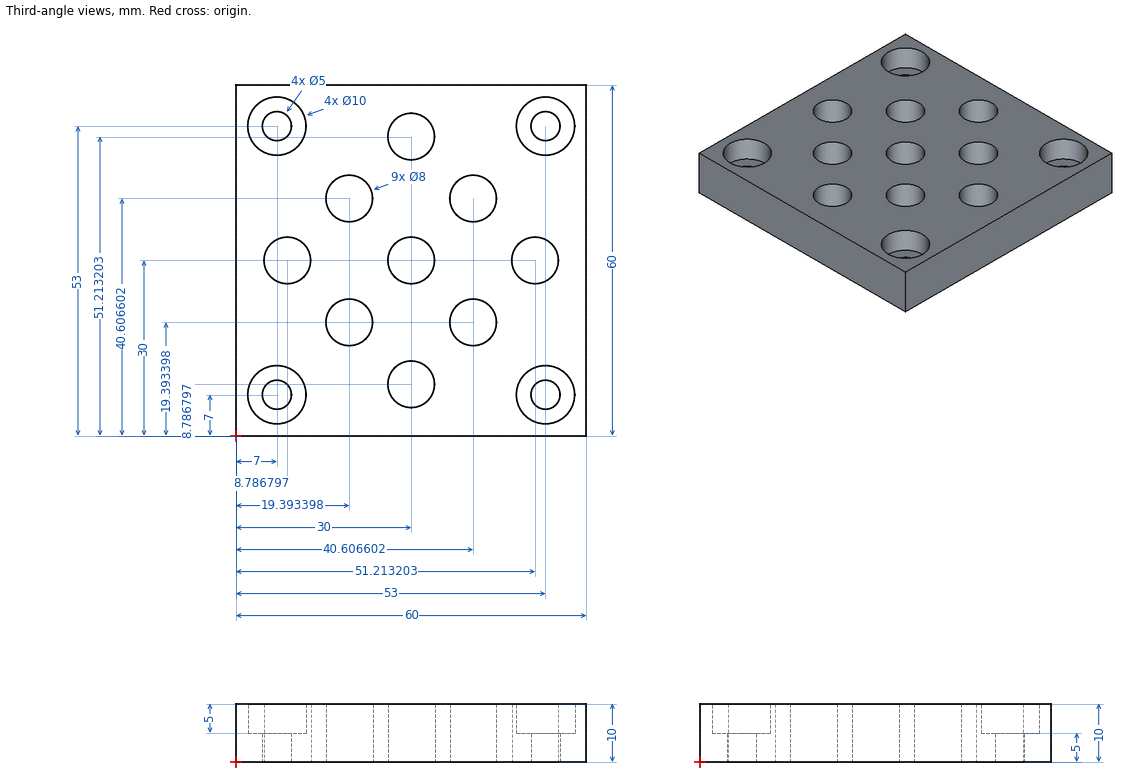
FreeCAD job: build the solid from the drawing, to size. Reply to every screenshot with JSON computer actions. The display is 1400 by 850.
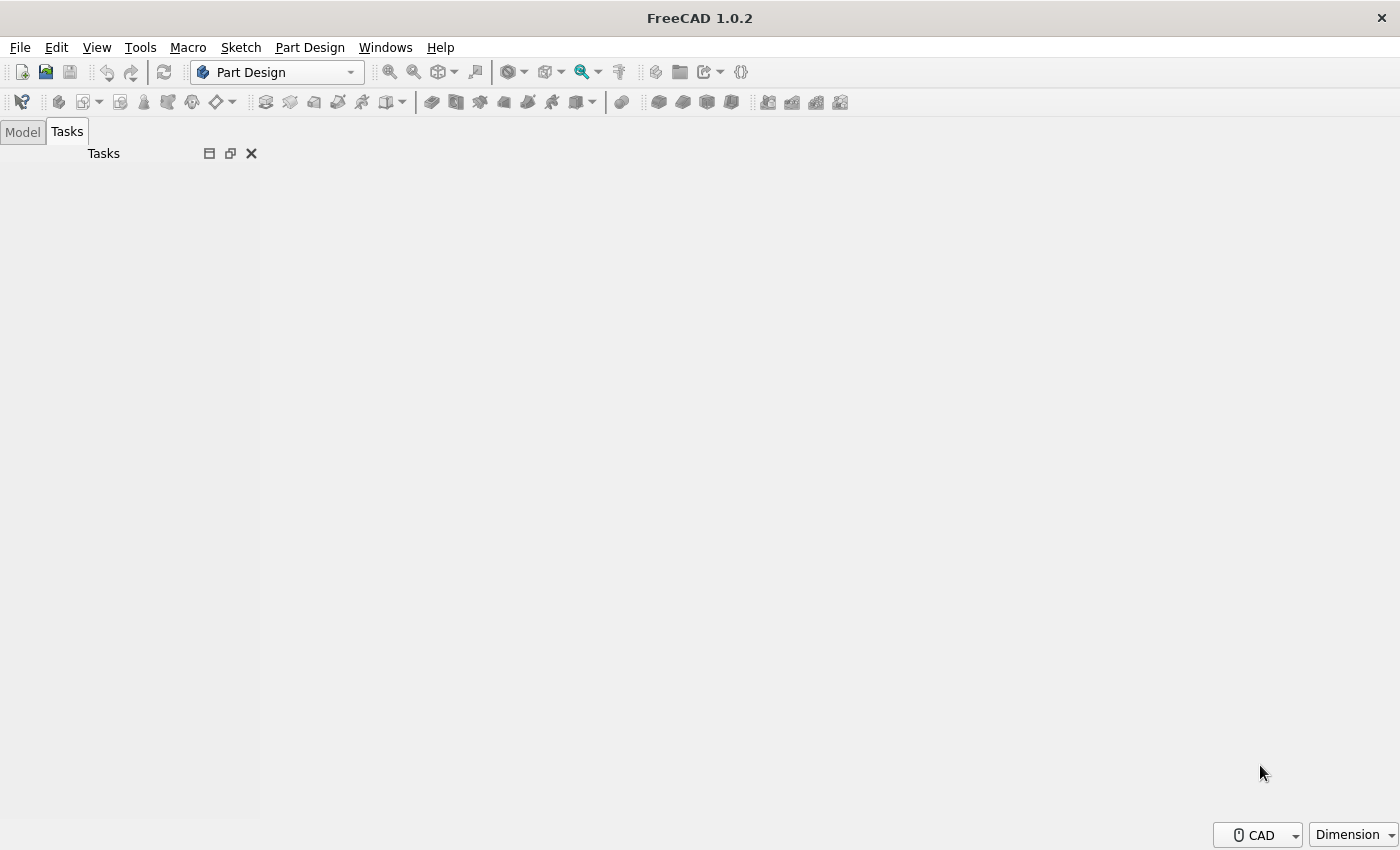
{"action": "left_click", "coordinate": [22, 72]}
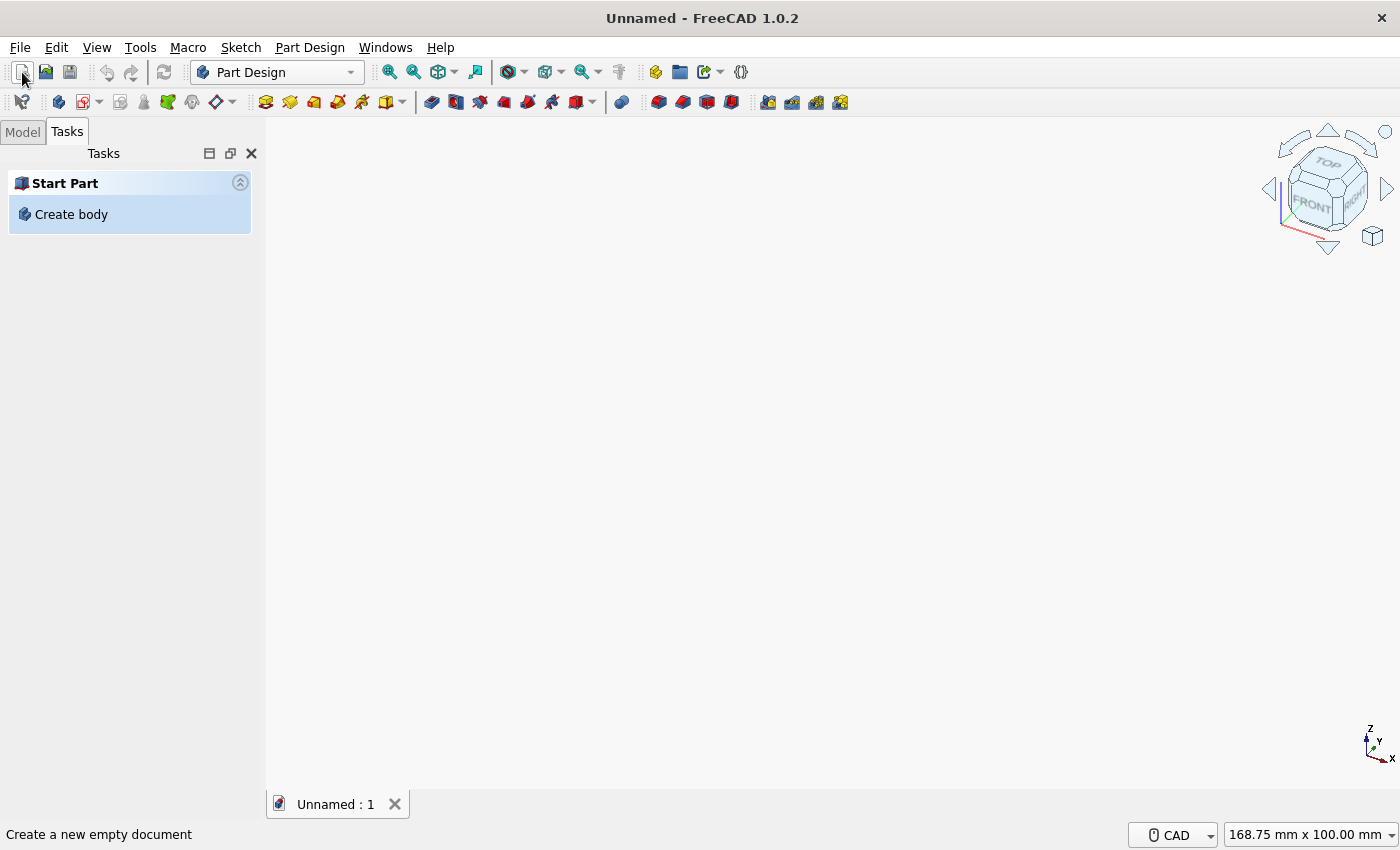
{"action": "left_click", "coordinate": [84, 102]}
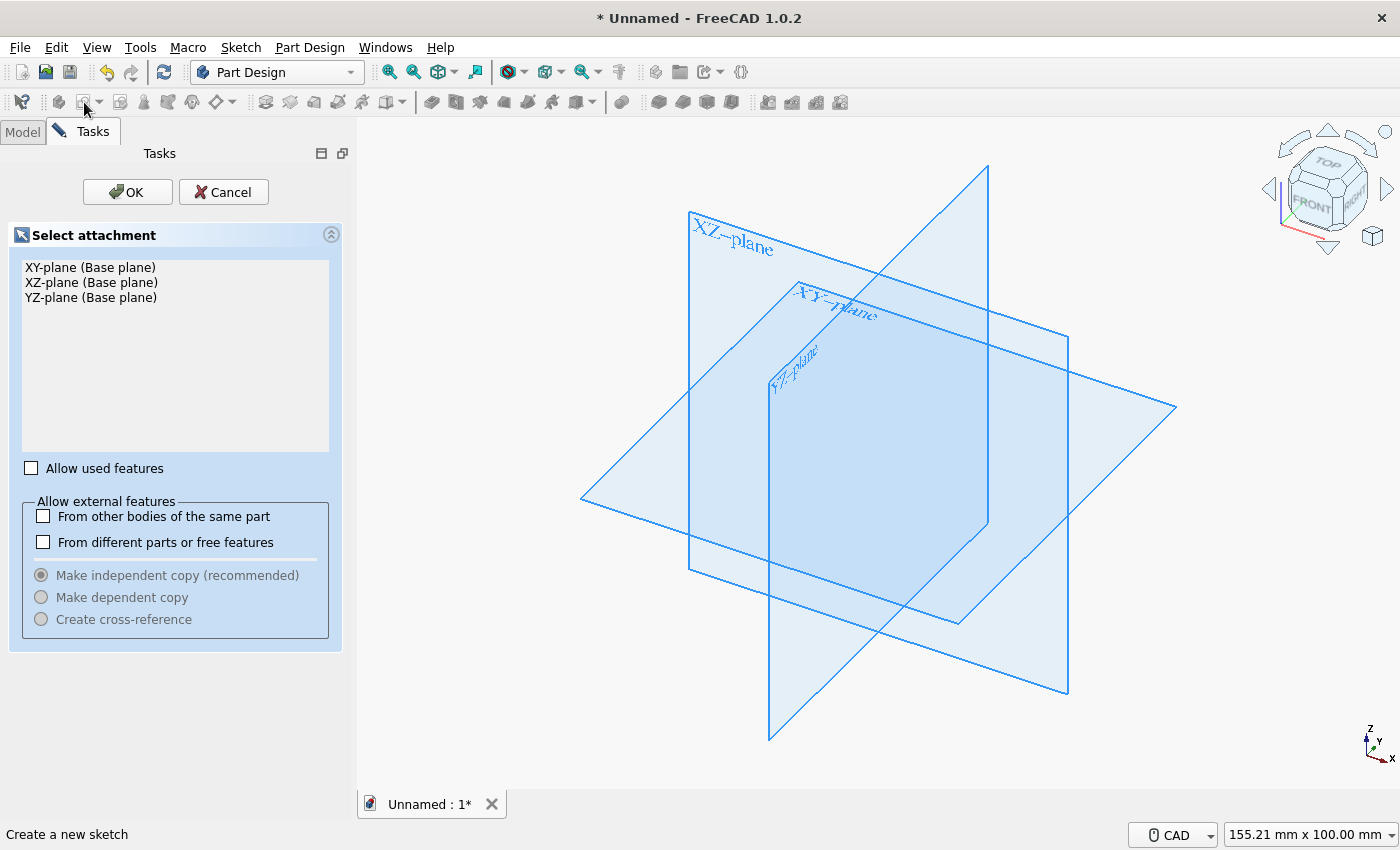
{"action": "left_click", "coordinate": [82, 268]}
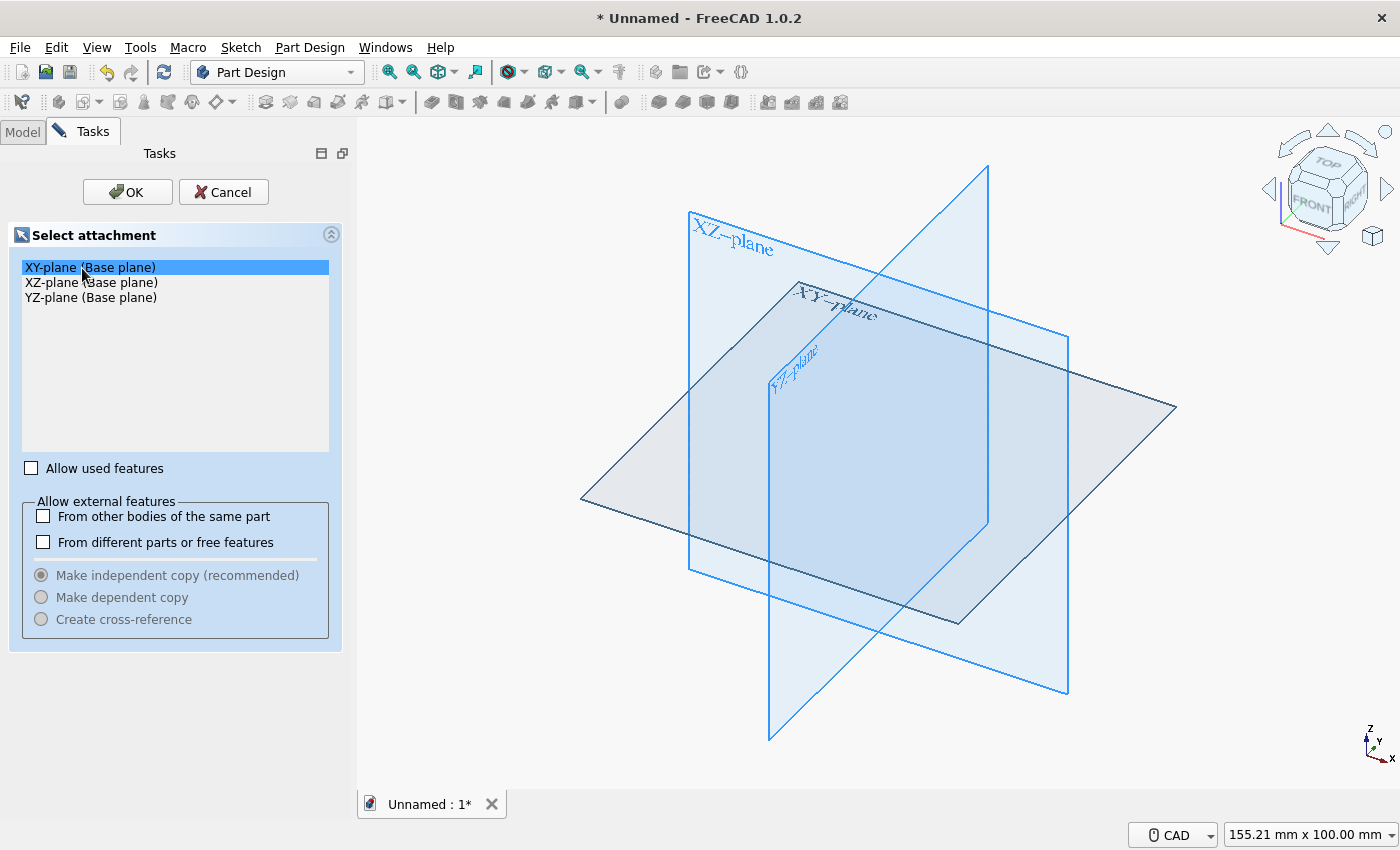
{"action": "left_click", "coordinate": [128, 192]}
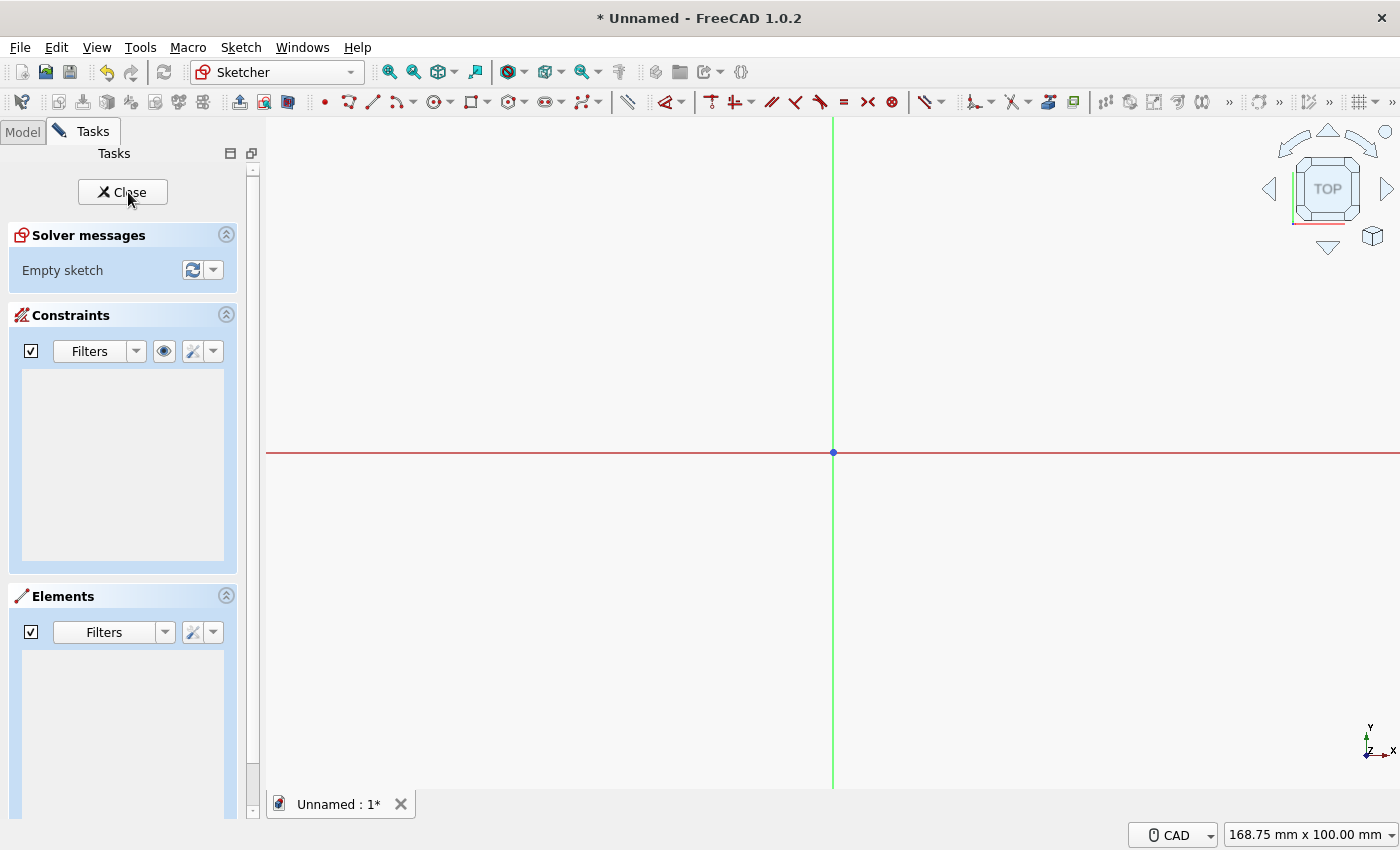
{"action": "scroll", "coordinate": [294, 761], "scroll_direction": "down", "scroll_amount": 1}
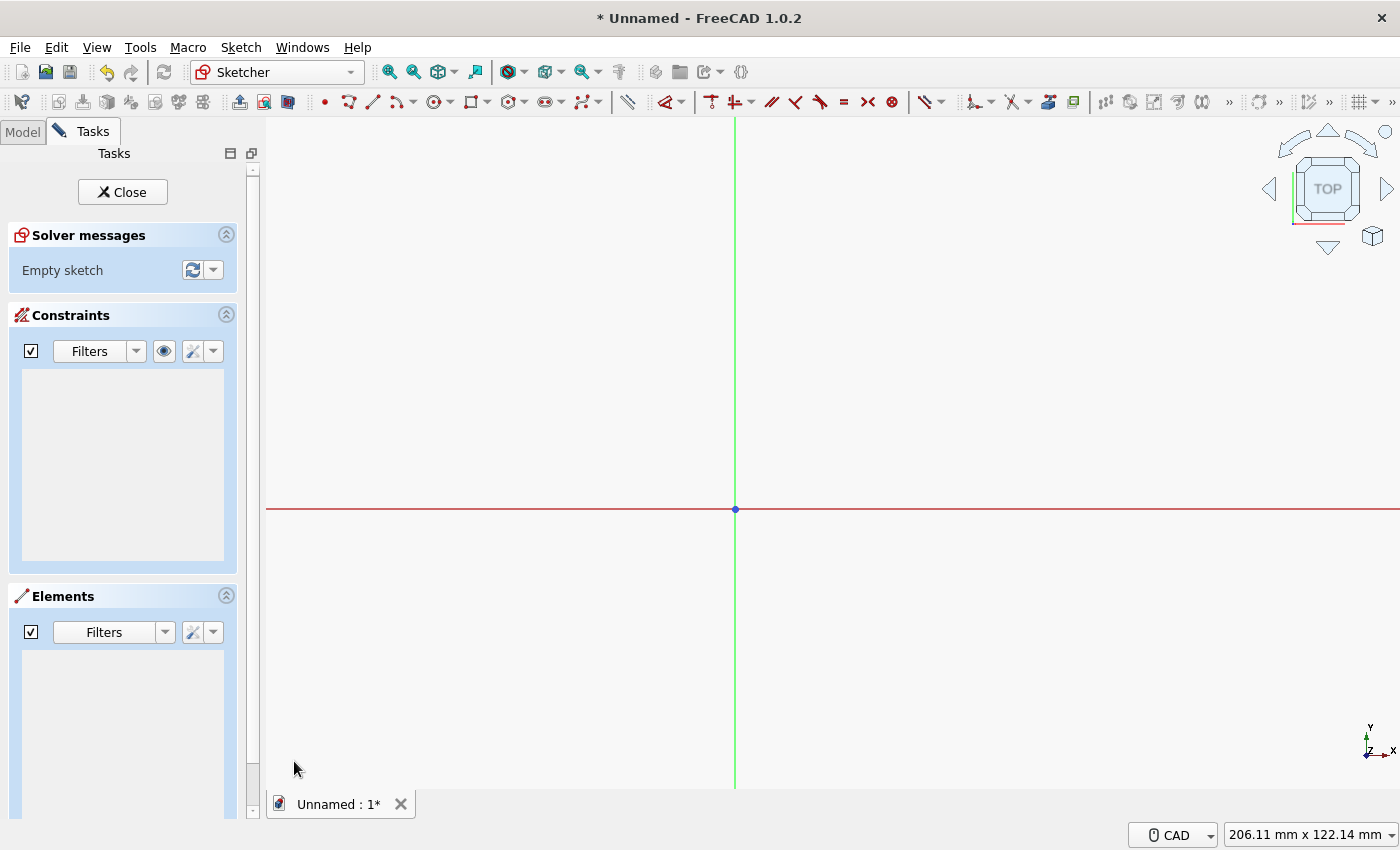
{"action": "left_click", "coordinate": [472, 102]}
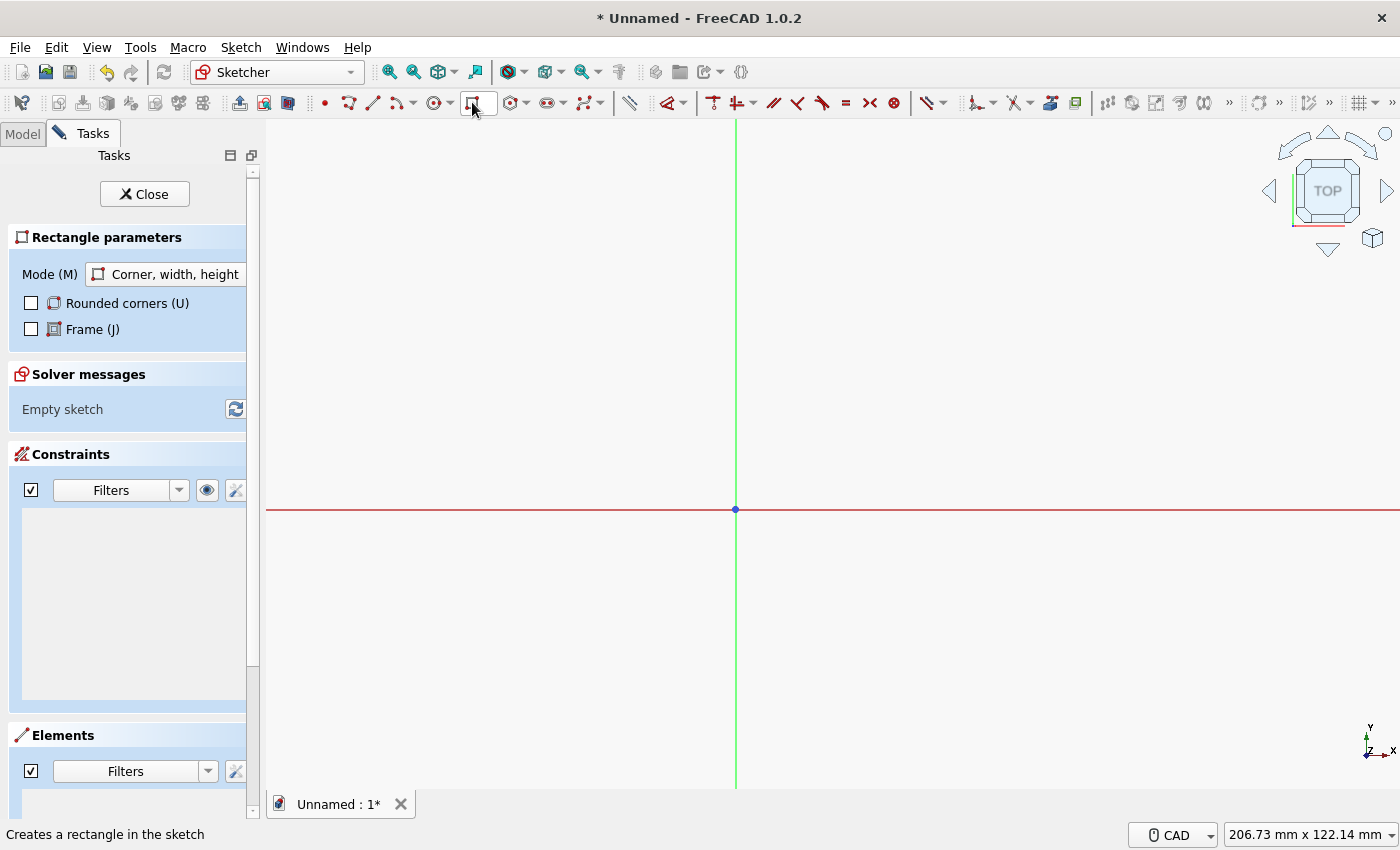
{"action": "left_click", "coordinate": [736, 510]}
{"action": "left_click", "coordinate": [1065, 181]}
{"action": "key", "text": "Escape"}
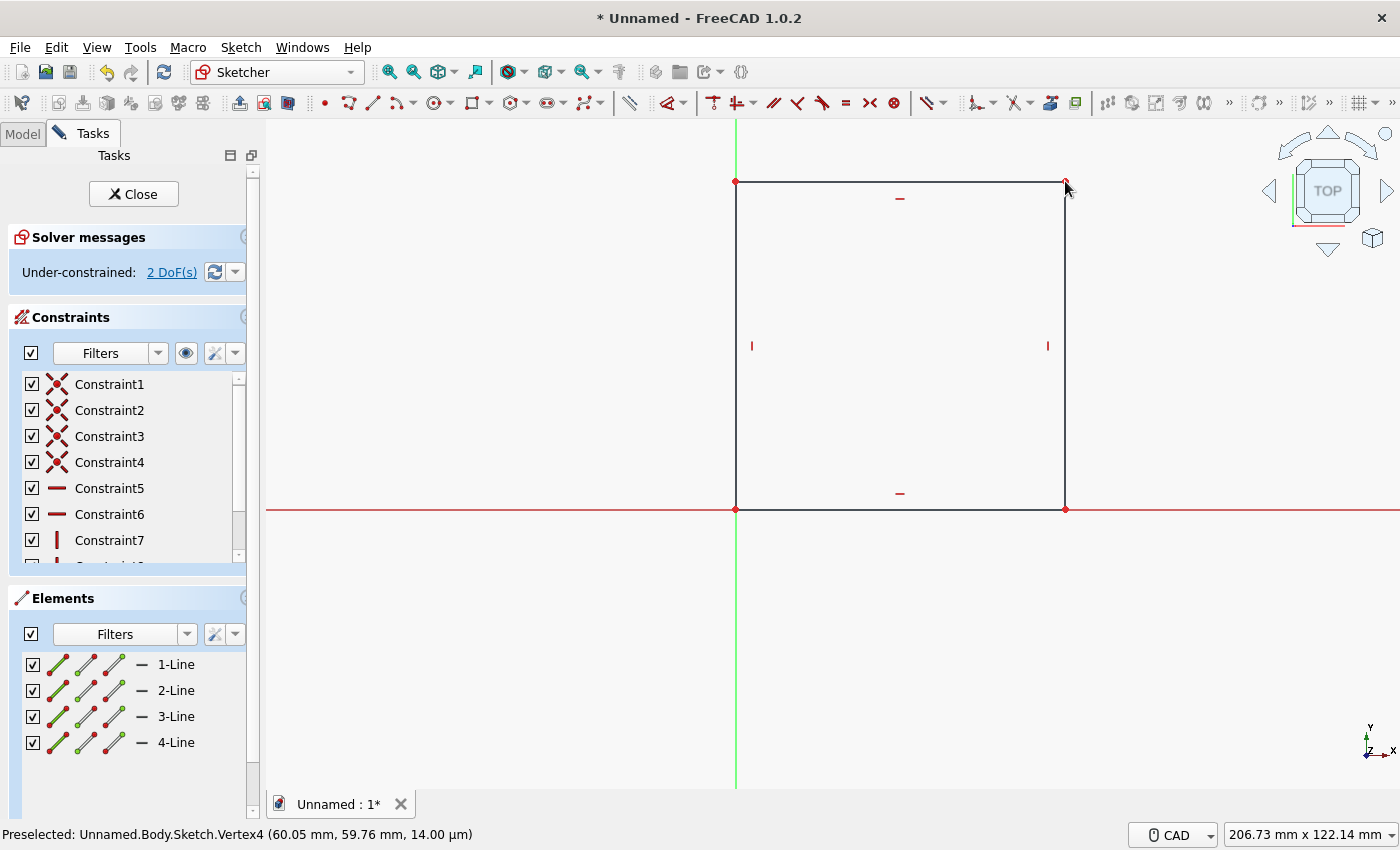
{"action": "left_click", "coordinate": [668, 104]}